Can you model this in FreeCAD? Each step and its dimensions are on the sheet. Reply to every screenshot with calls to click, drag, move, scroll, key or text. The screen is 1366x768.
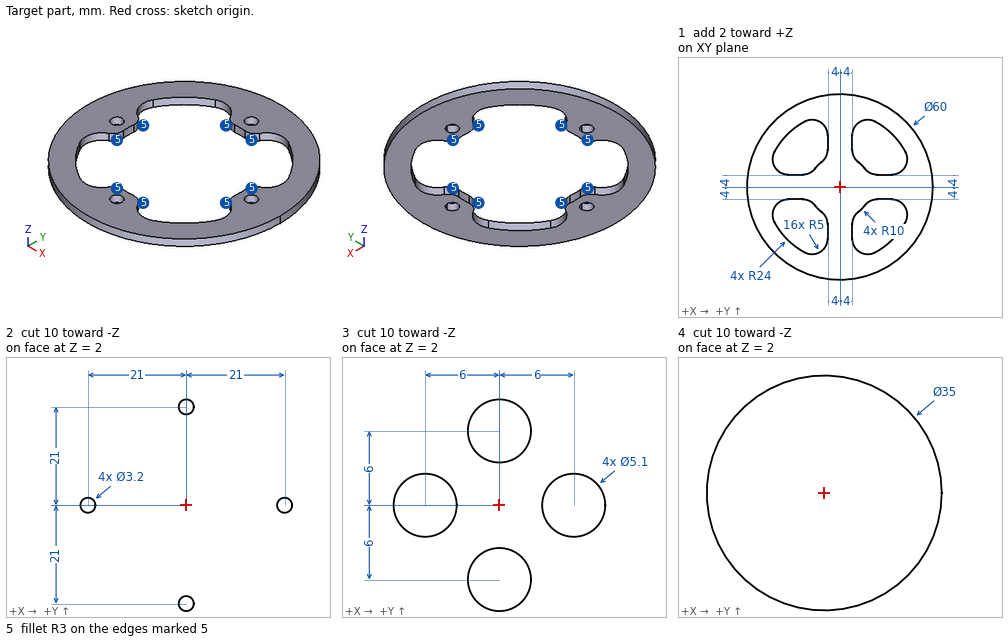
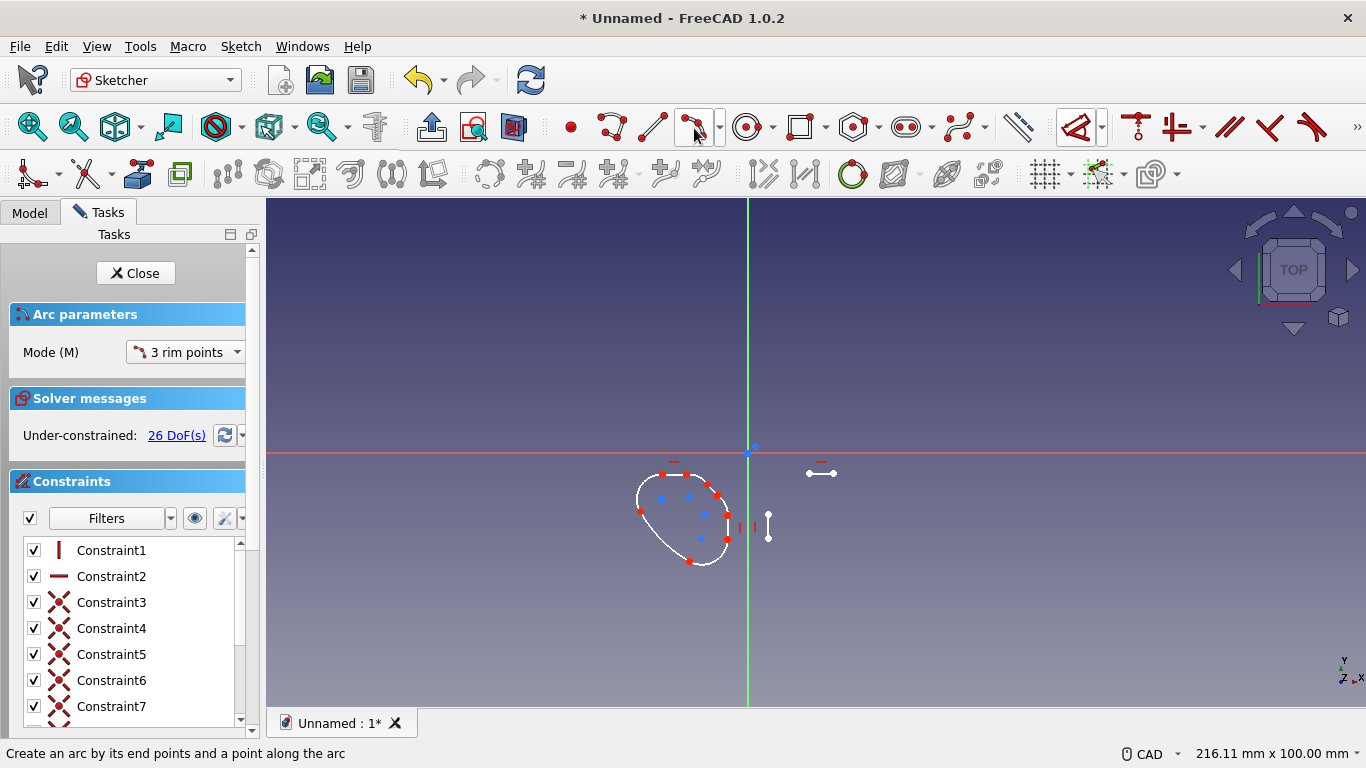
scroll(833, 473, up, 2)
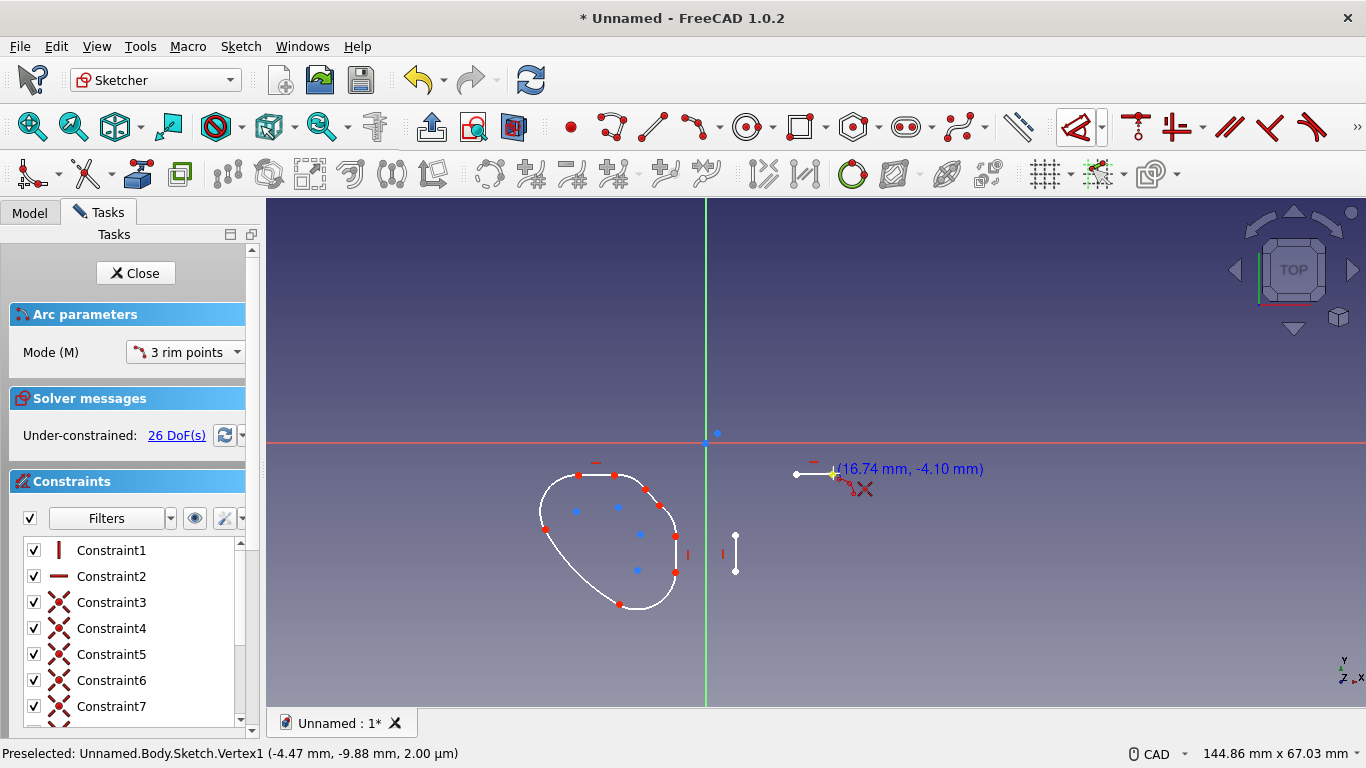
click(833, 474)
click(866, 529)
click(865, 492)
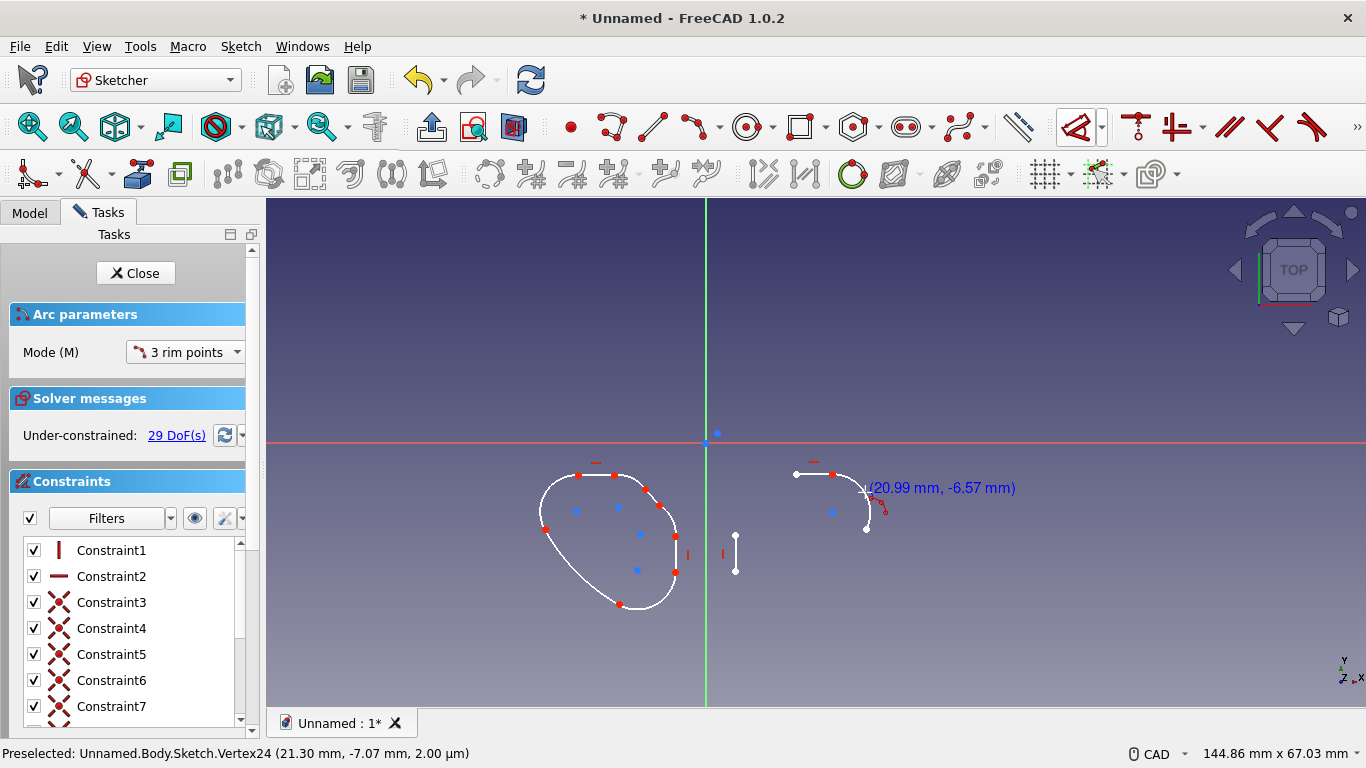
click(866, 530)
click(792, 604)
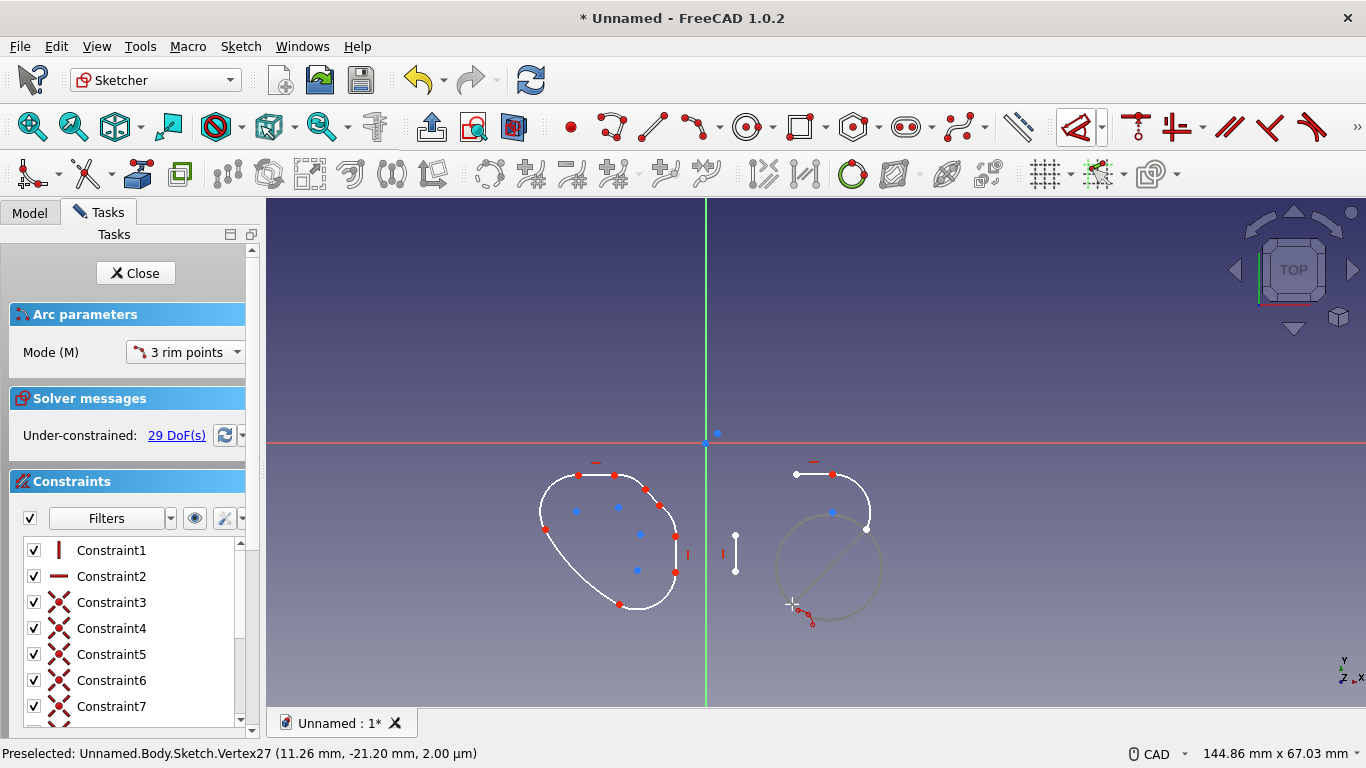
scroll(834, 572, up, 4)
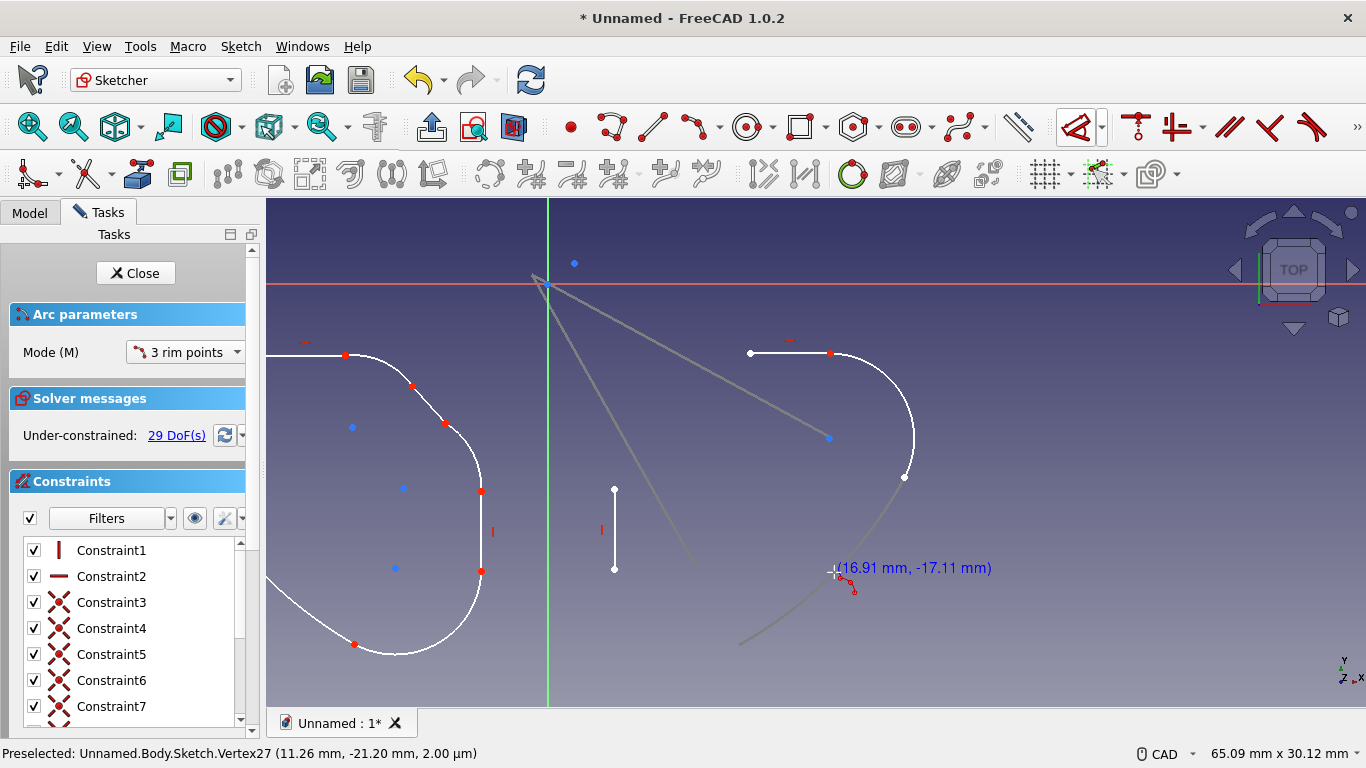
click(834, 571)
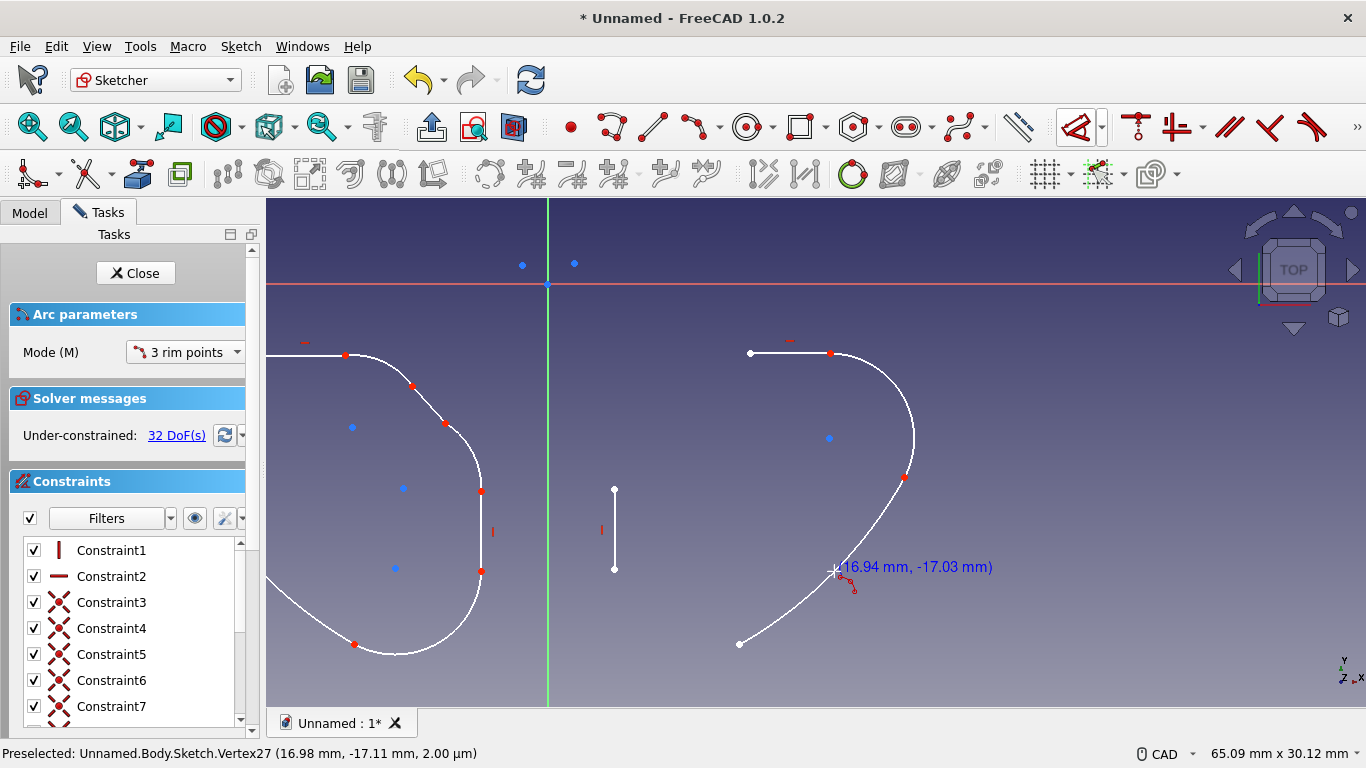
click(740, 645)
click(615, 569)
click(656, 640)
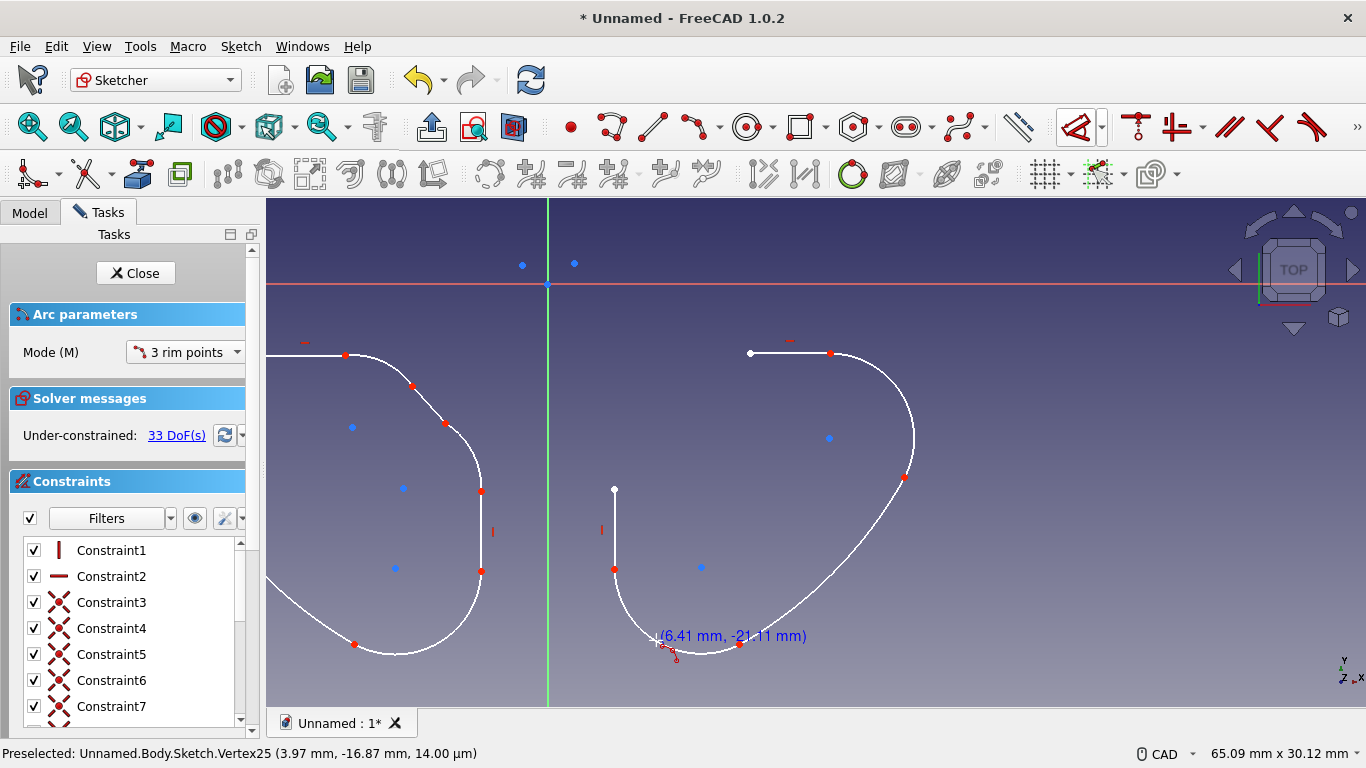
click(615, 490)
click(649, 419)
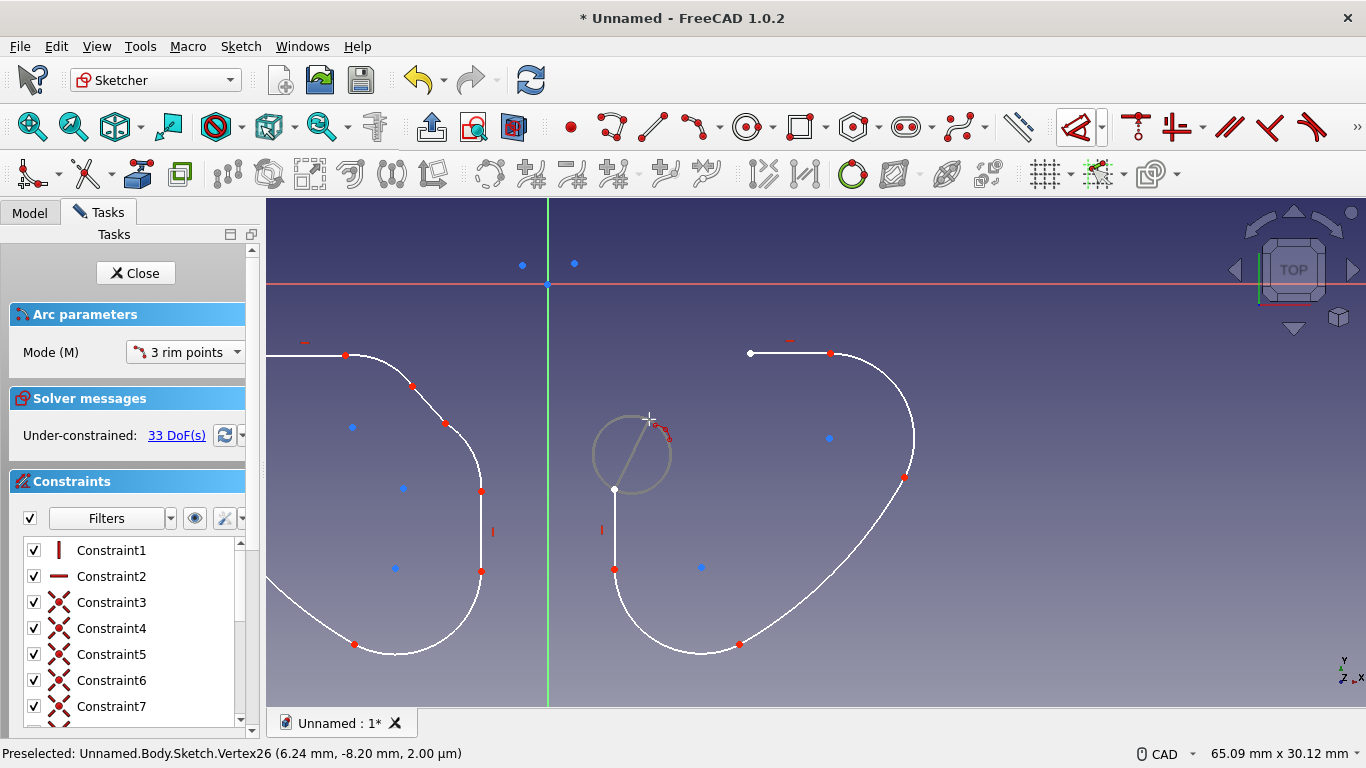
scroll(624, 449, up, 3)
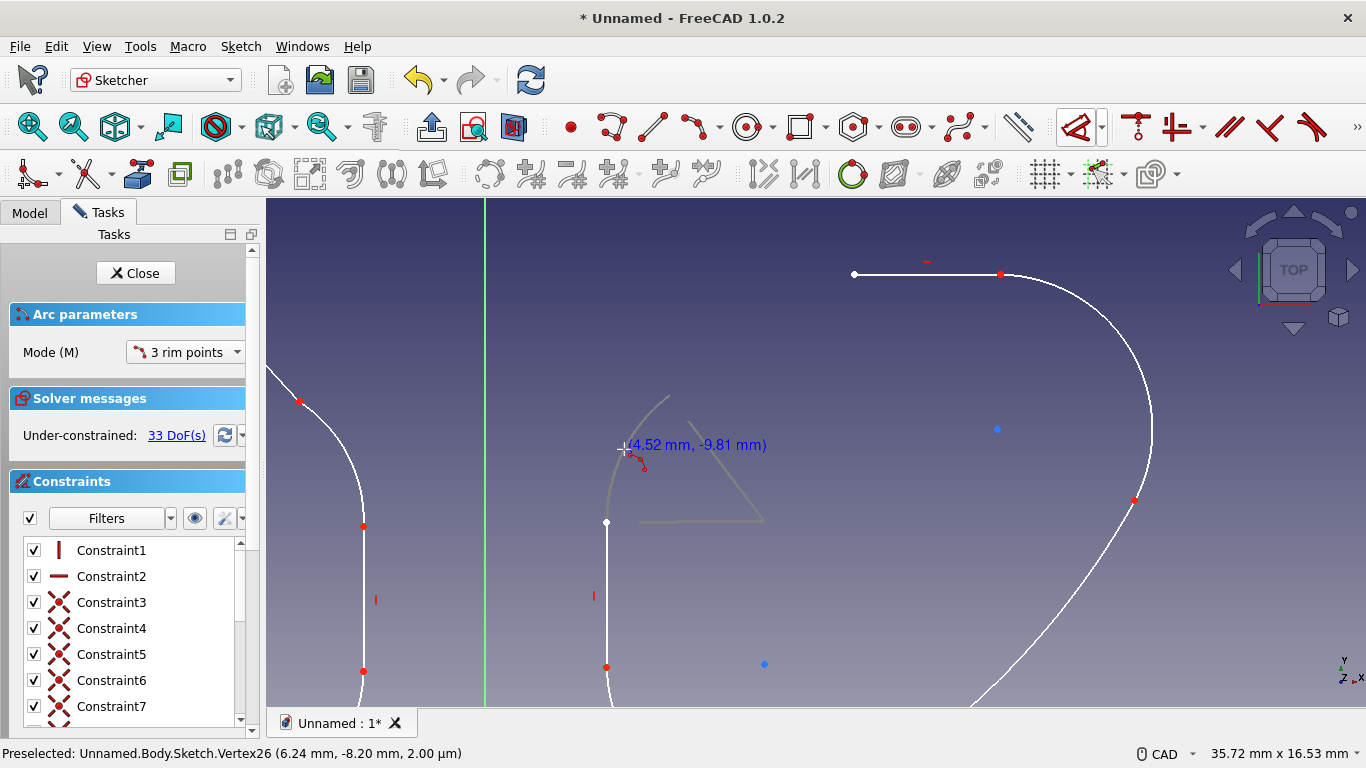
click(624, 449)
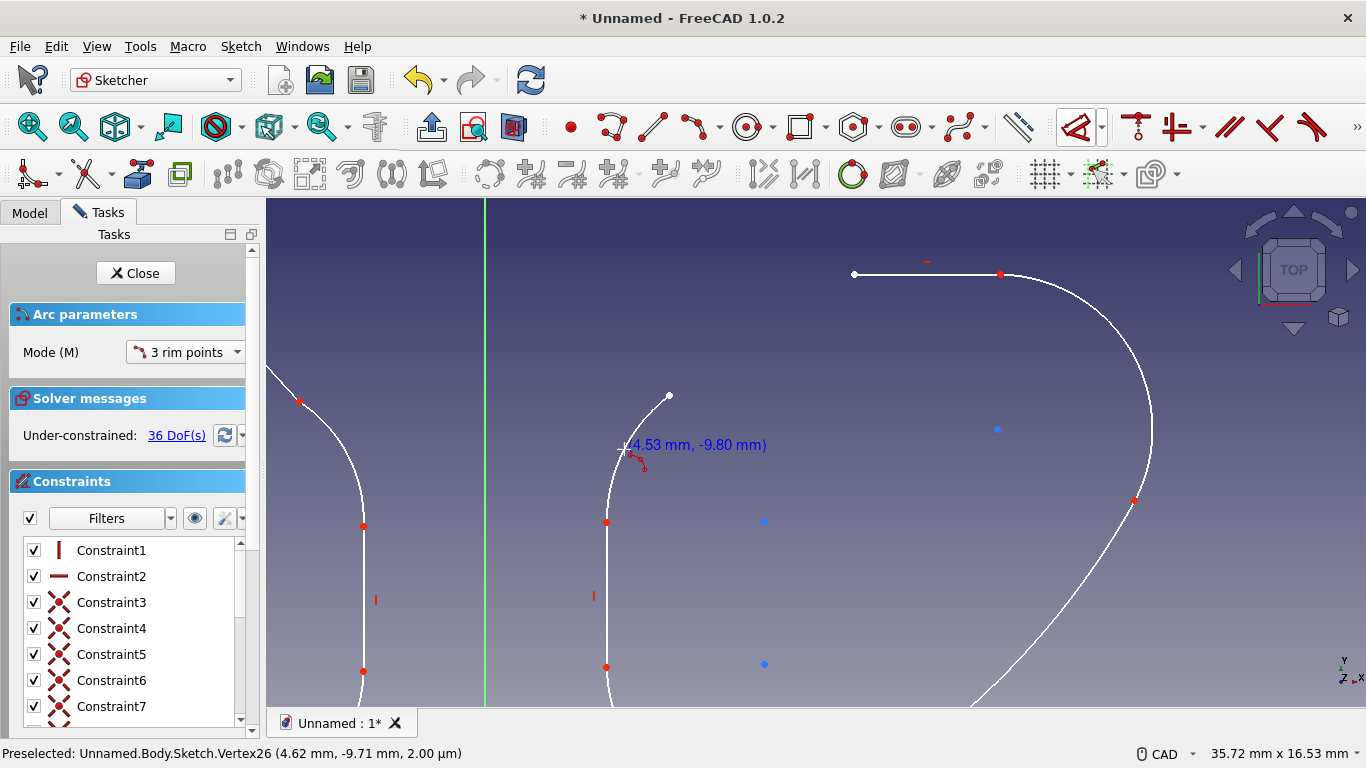
scroll(800, 513, down, 9)